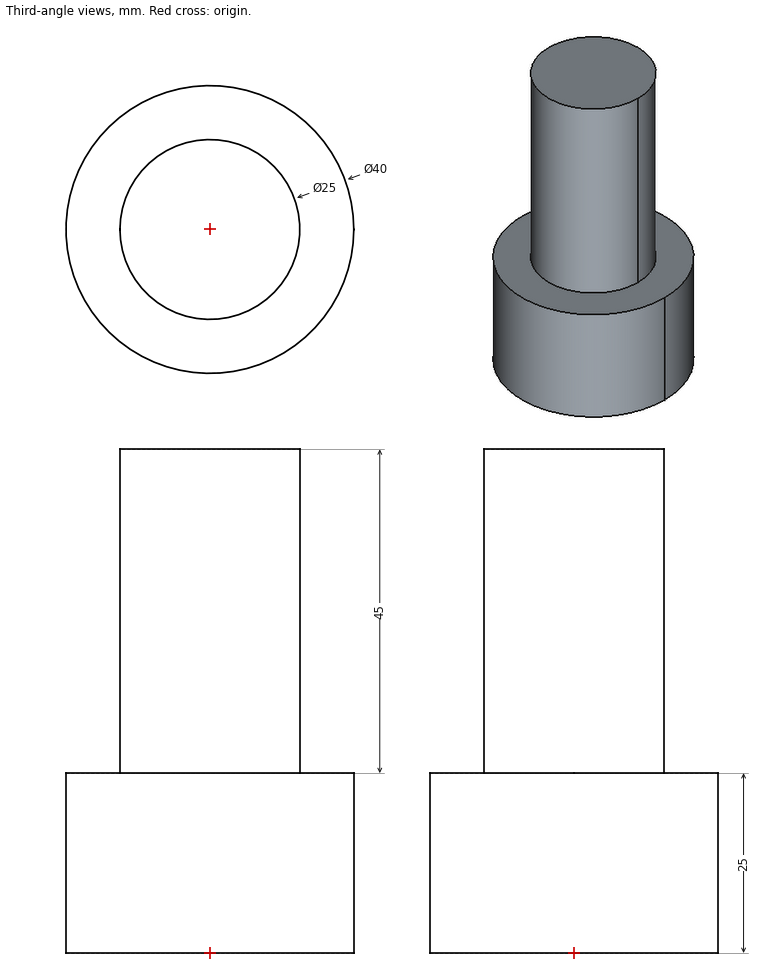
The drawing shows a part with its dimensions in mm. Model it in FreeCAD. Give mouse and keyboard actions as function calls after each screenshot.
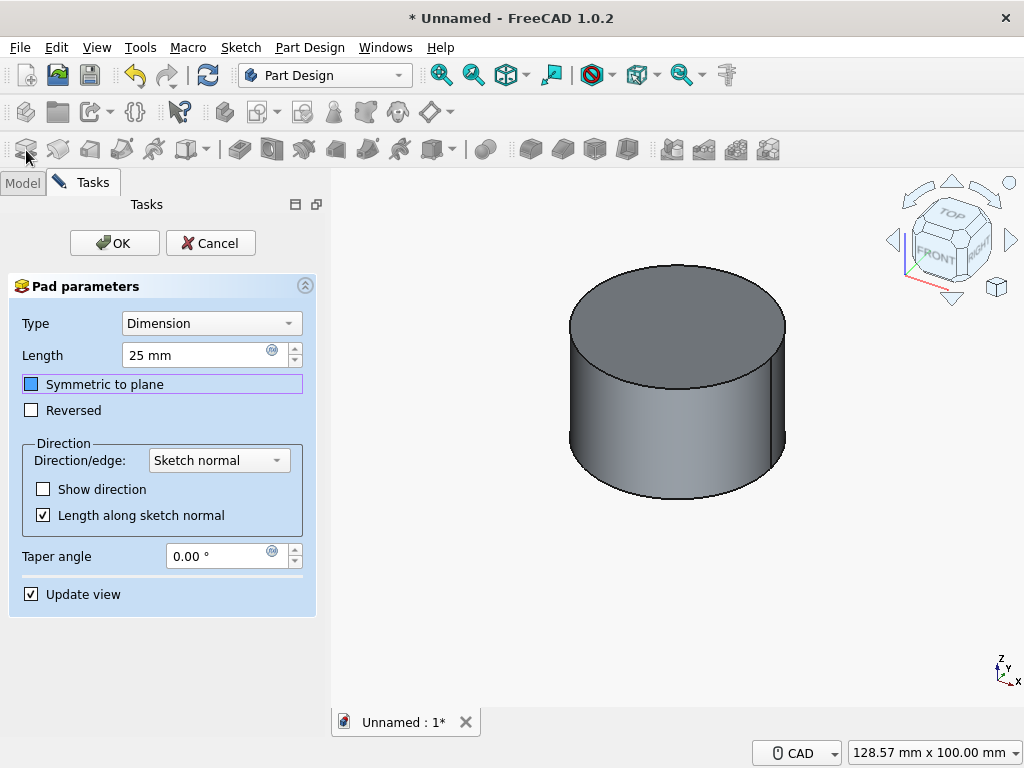
click(115, 243)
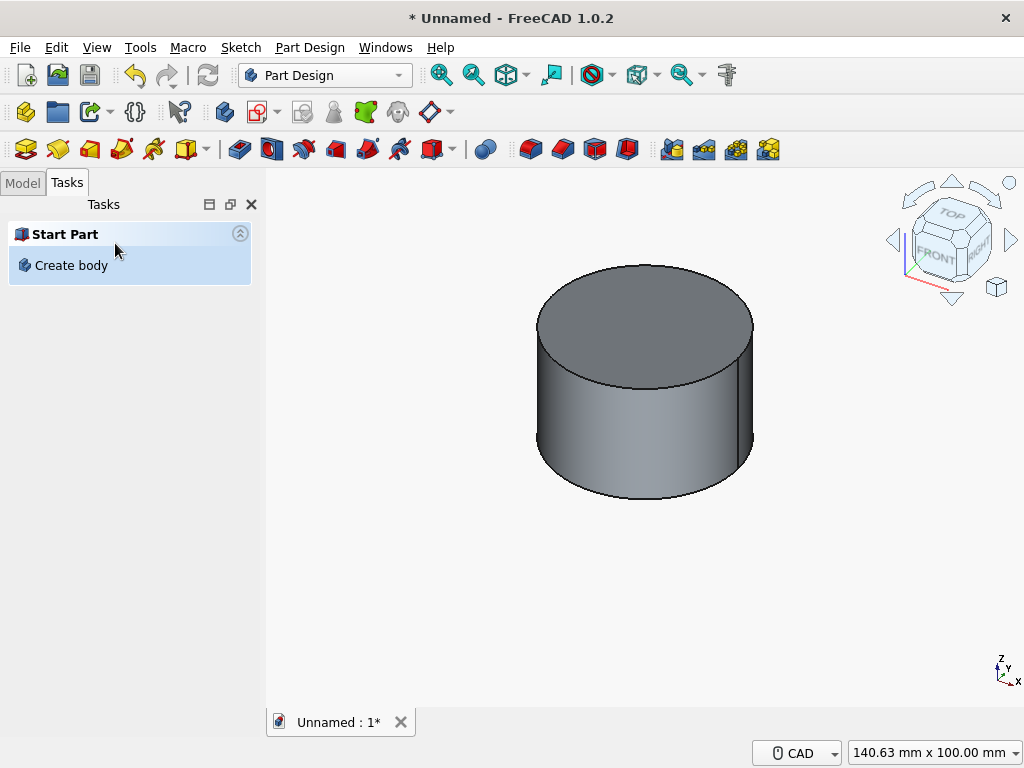
click(645, 326)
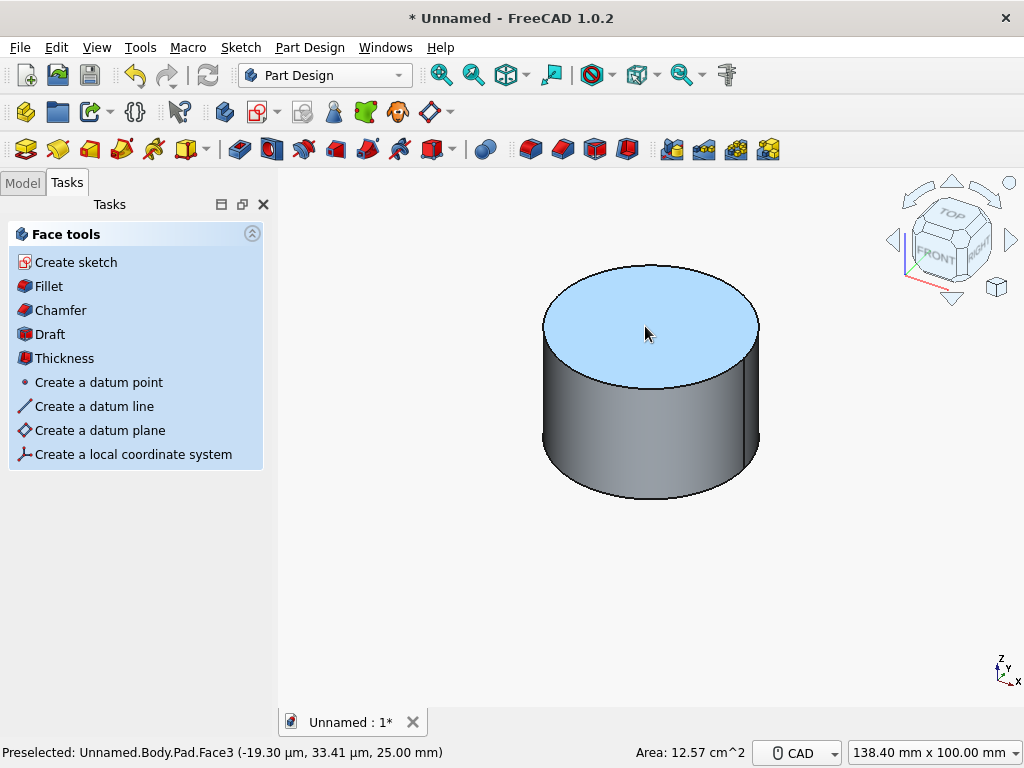
click(258, 112)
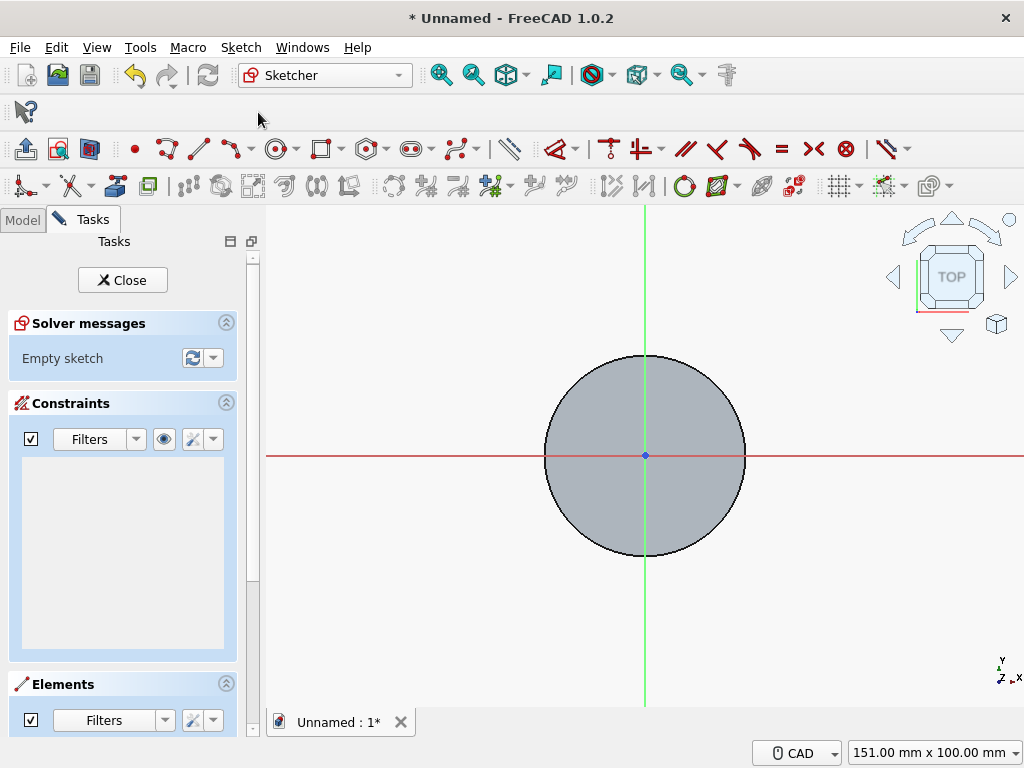
scroll(685, 456, up, 5)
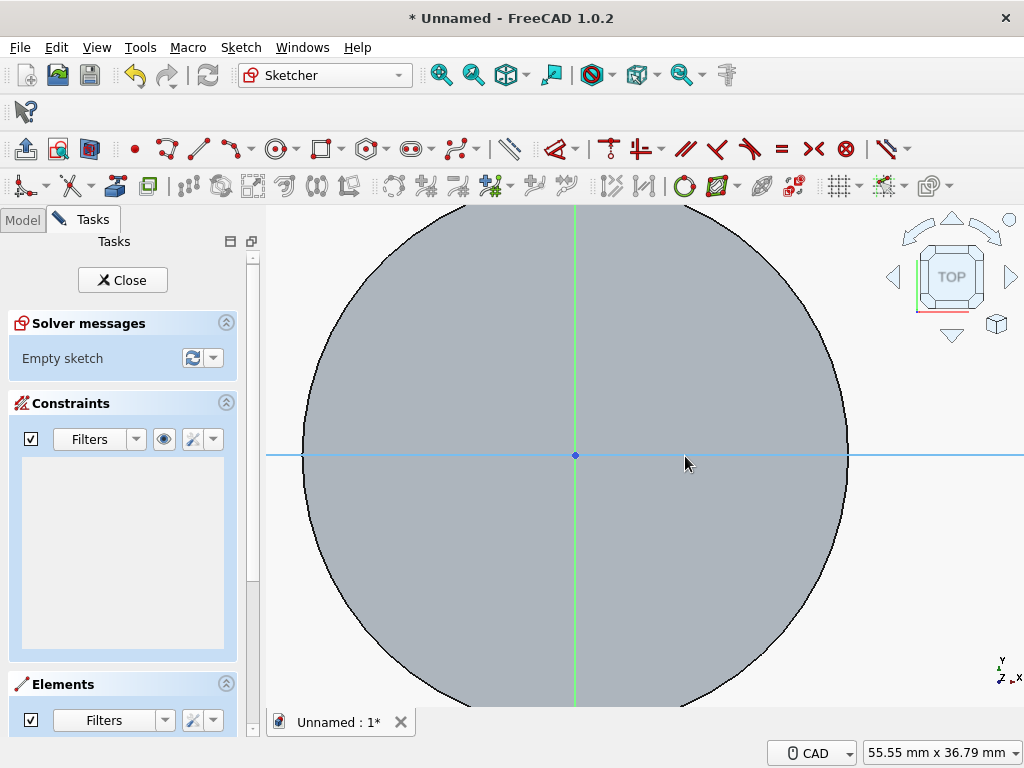
click(276, 150)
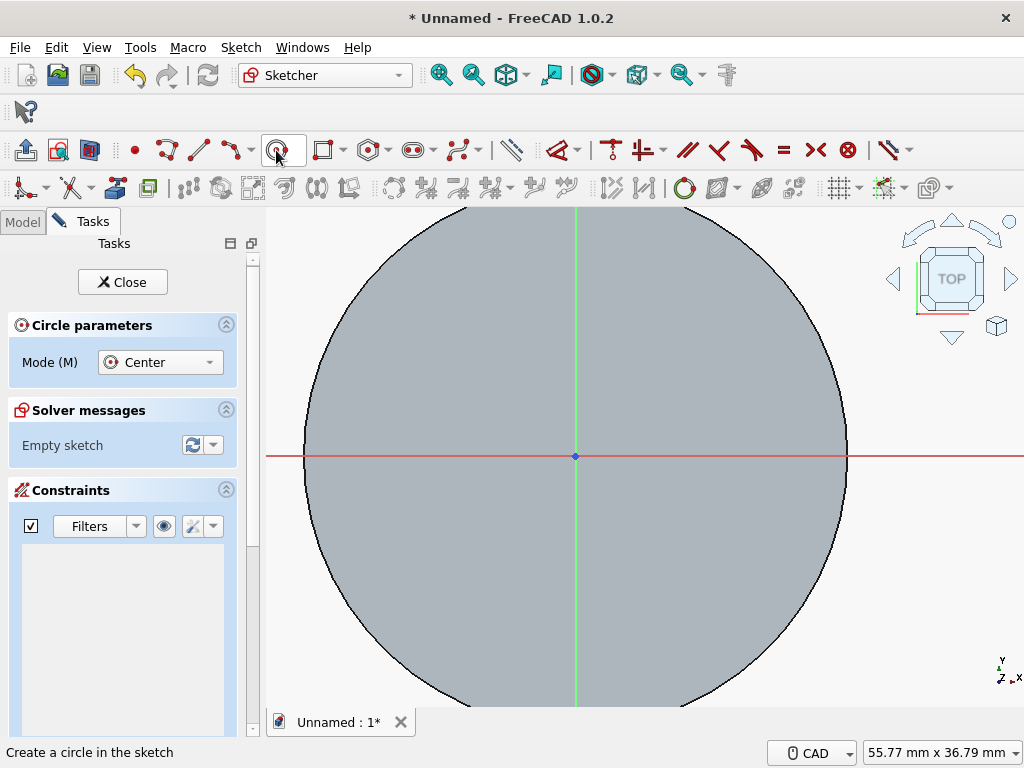
click(576, 456)
click(696, 336)
key(Escape)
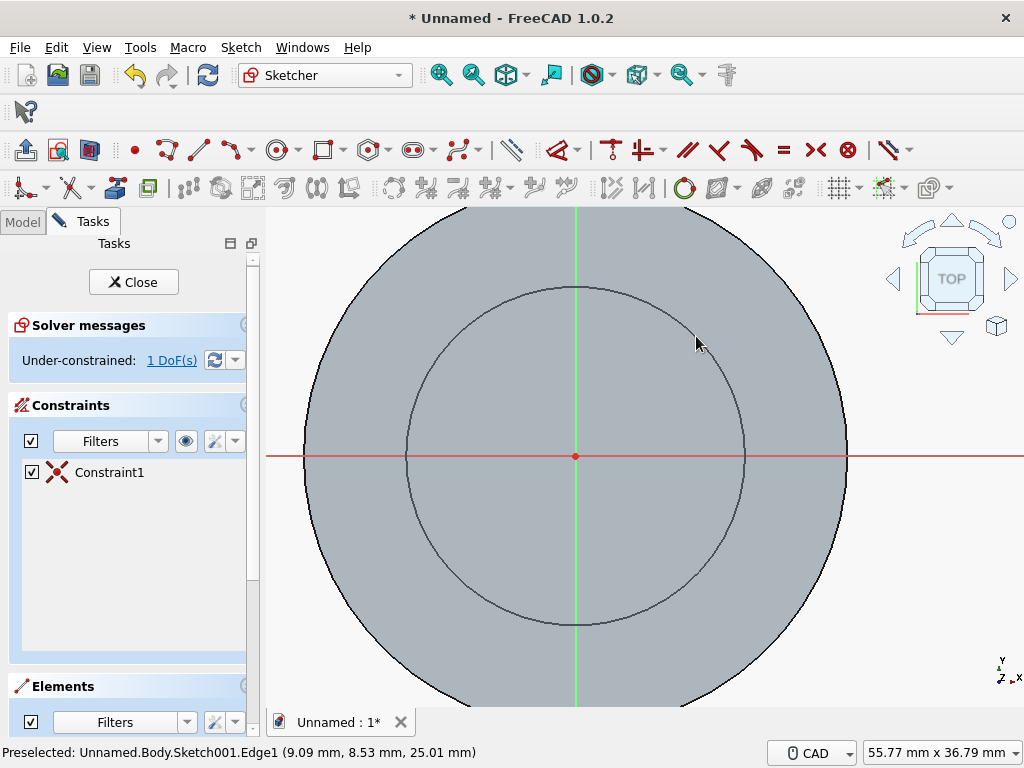
click(695, 336)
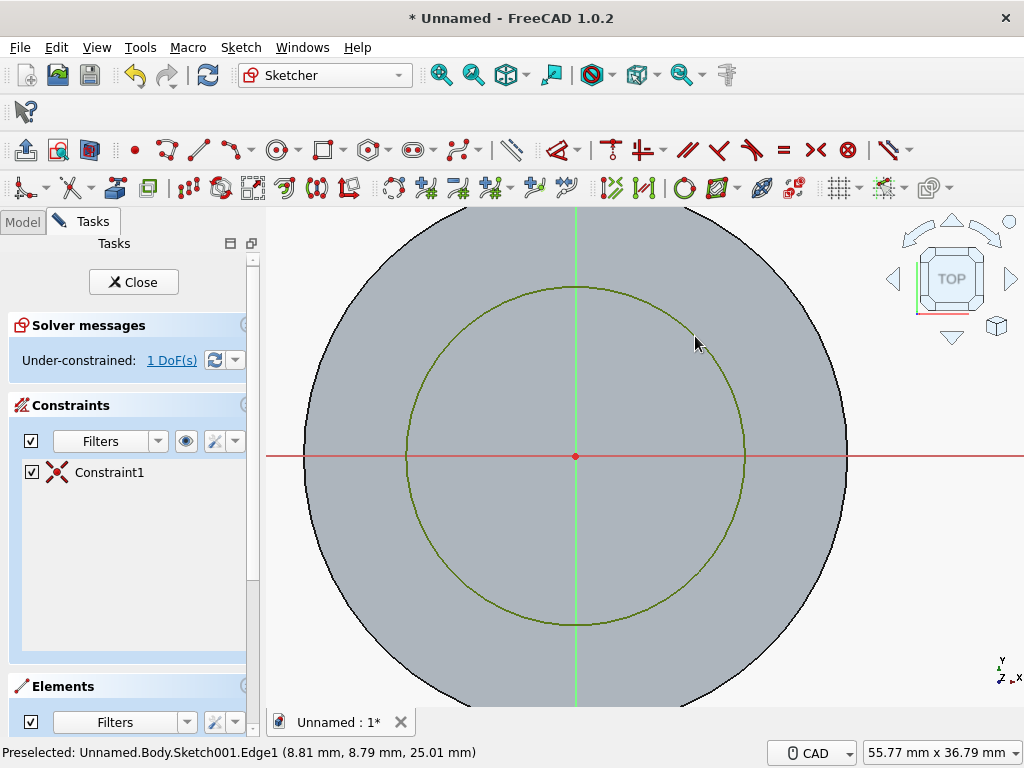
click(580, 150)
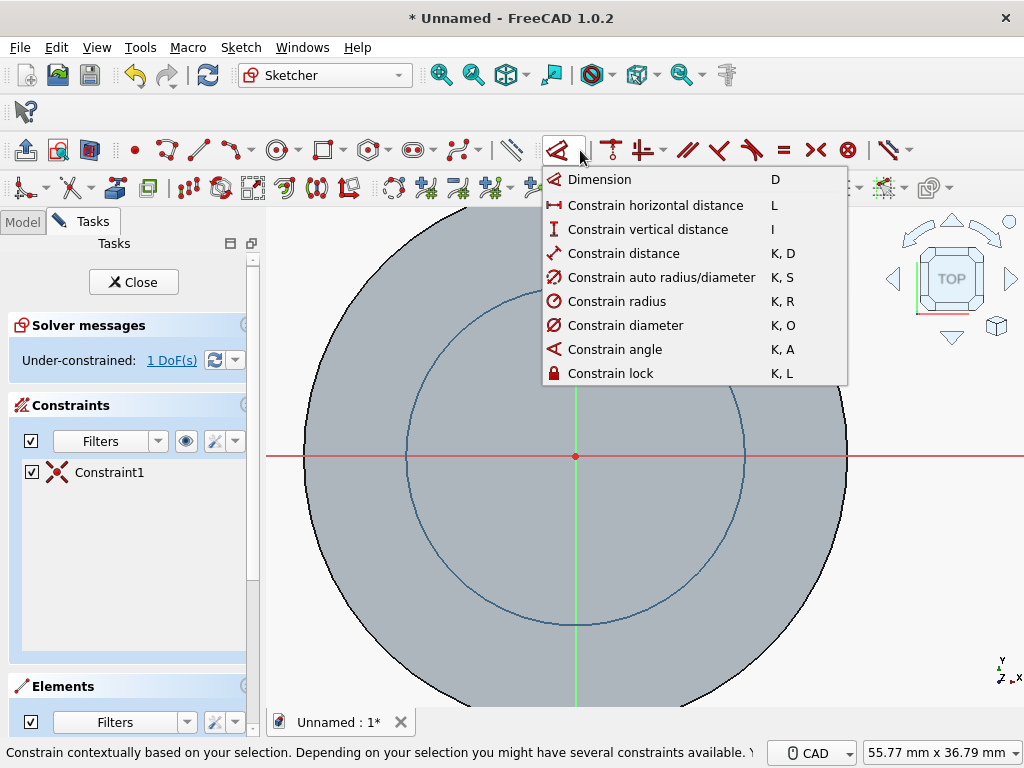
click(695, 325)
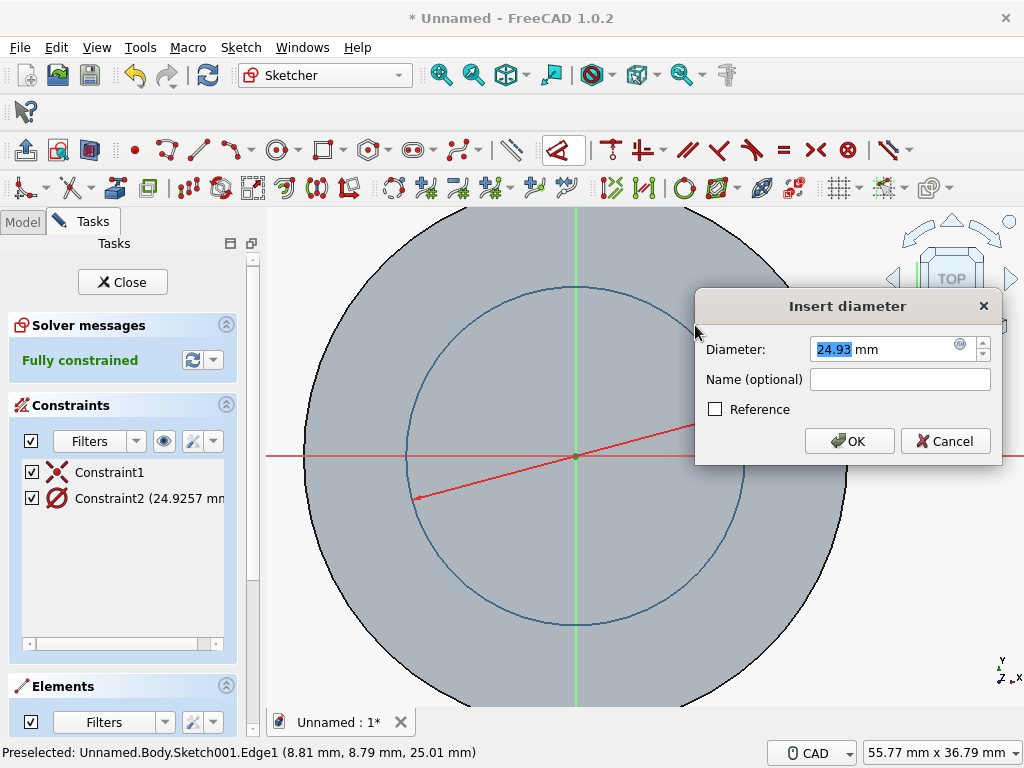
text(25)
key(Return)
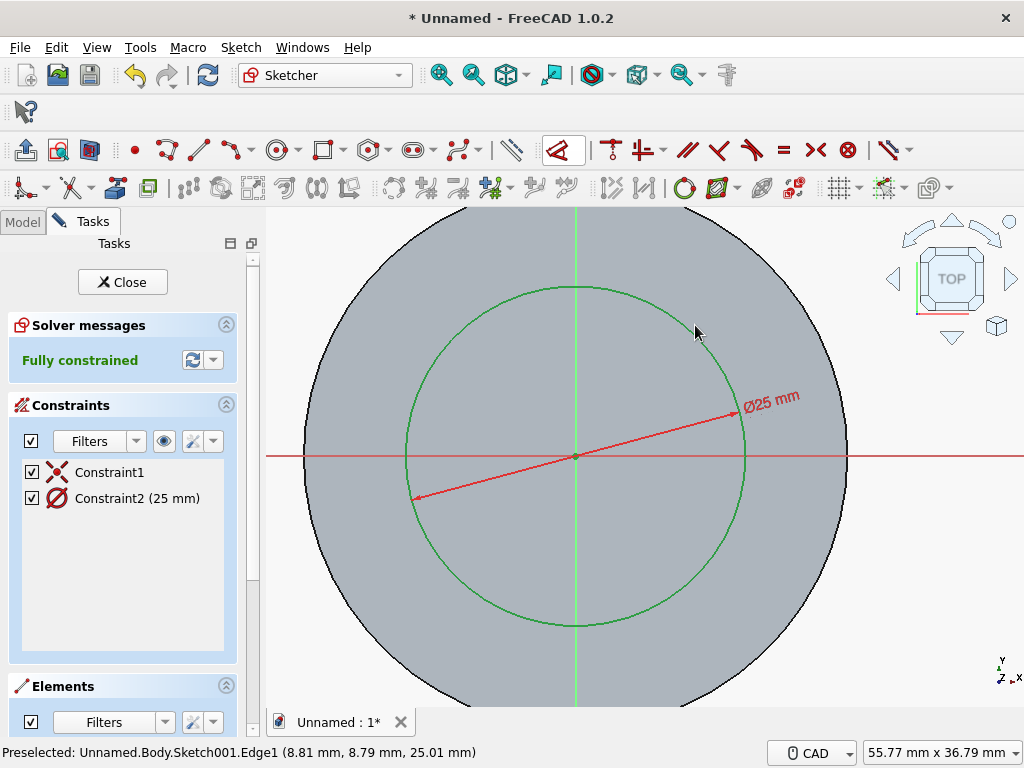
click(123, 282)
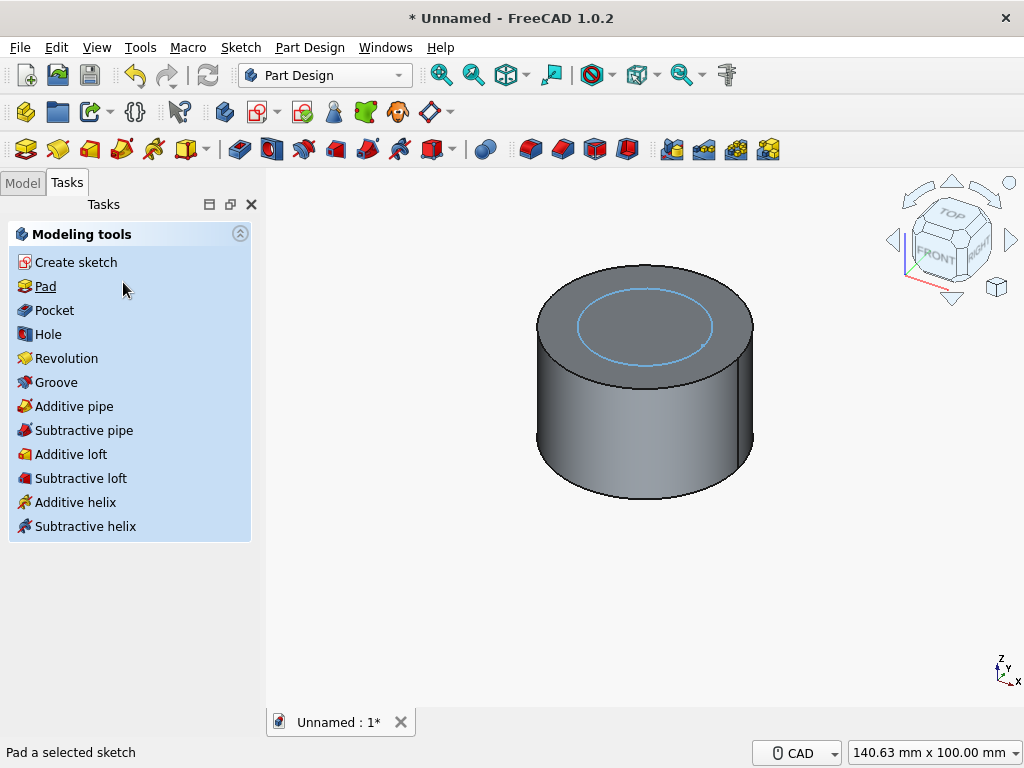
click(26, 150)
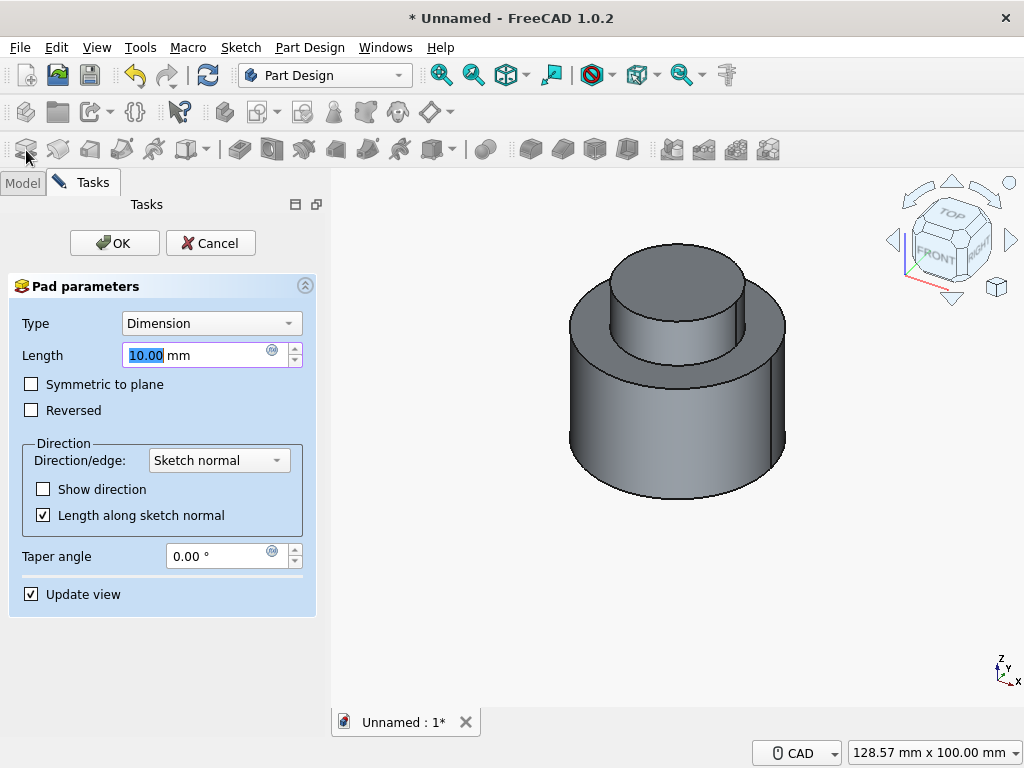
text(45)
key(Tab)